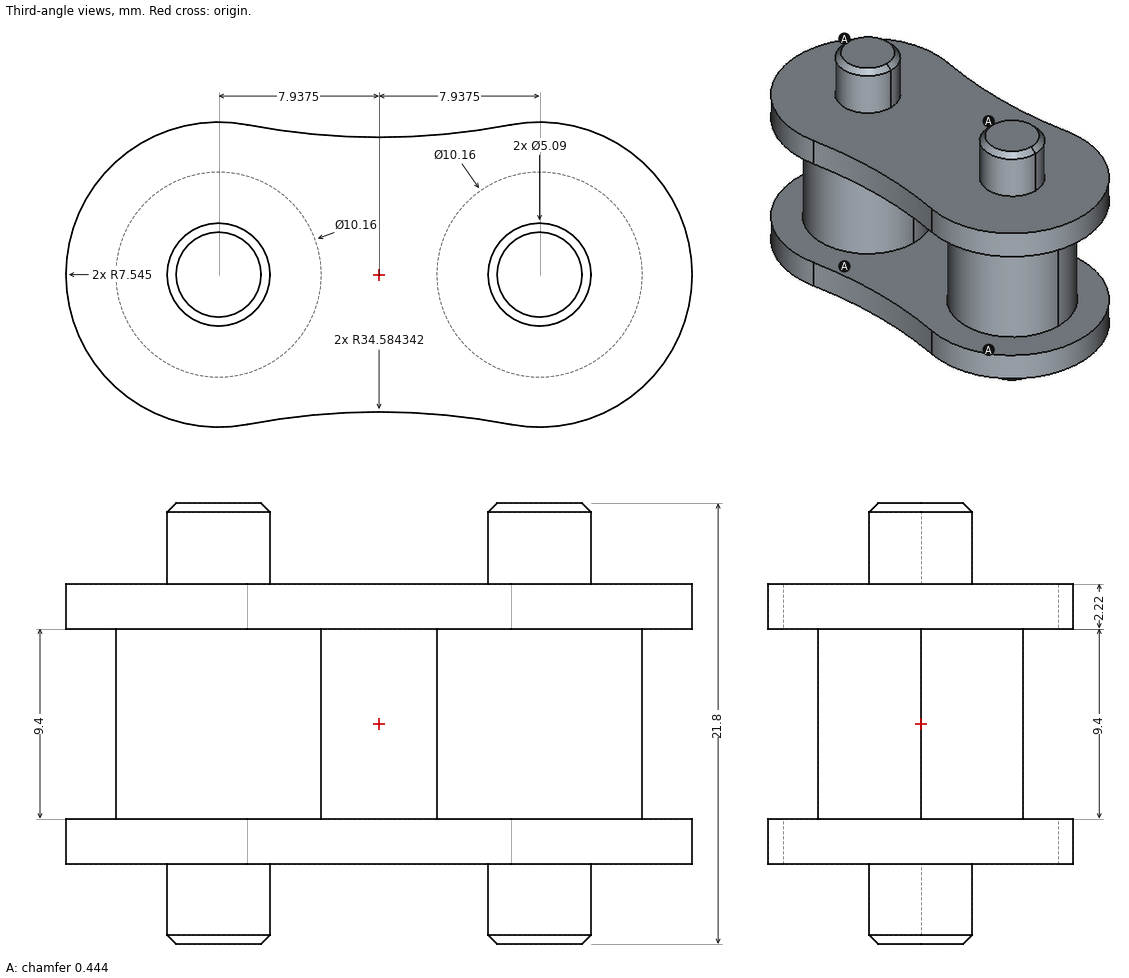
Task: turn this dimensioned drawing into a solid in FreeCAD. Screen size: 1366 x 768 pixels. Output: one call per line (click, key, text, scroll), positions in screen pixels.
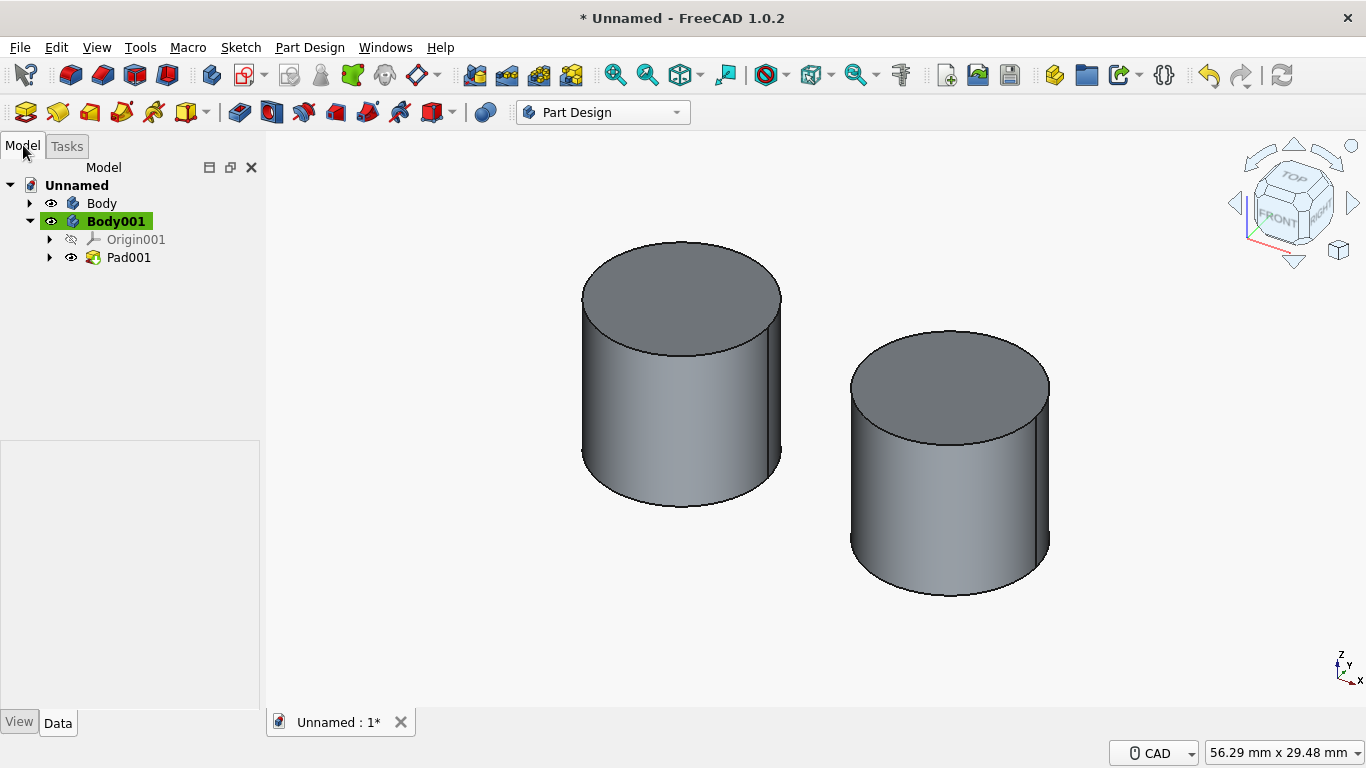
double_click(96, 203)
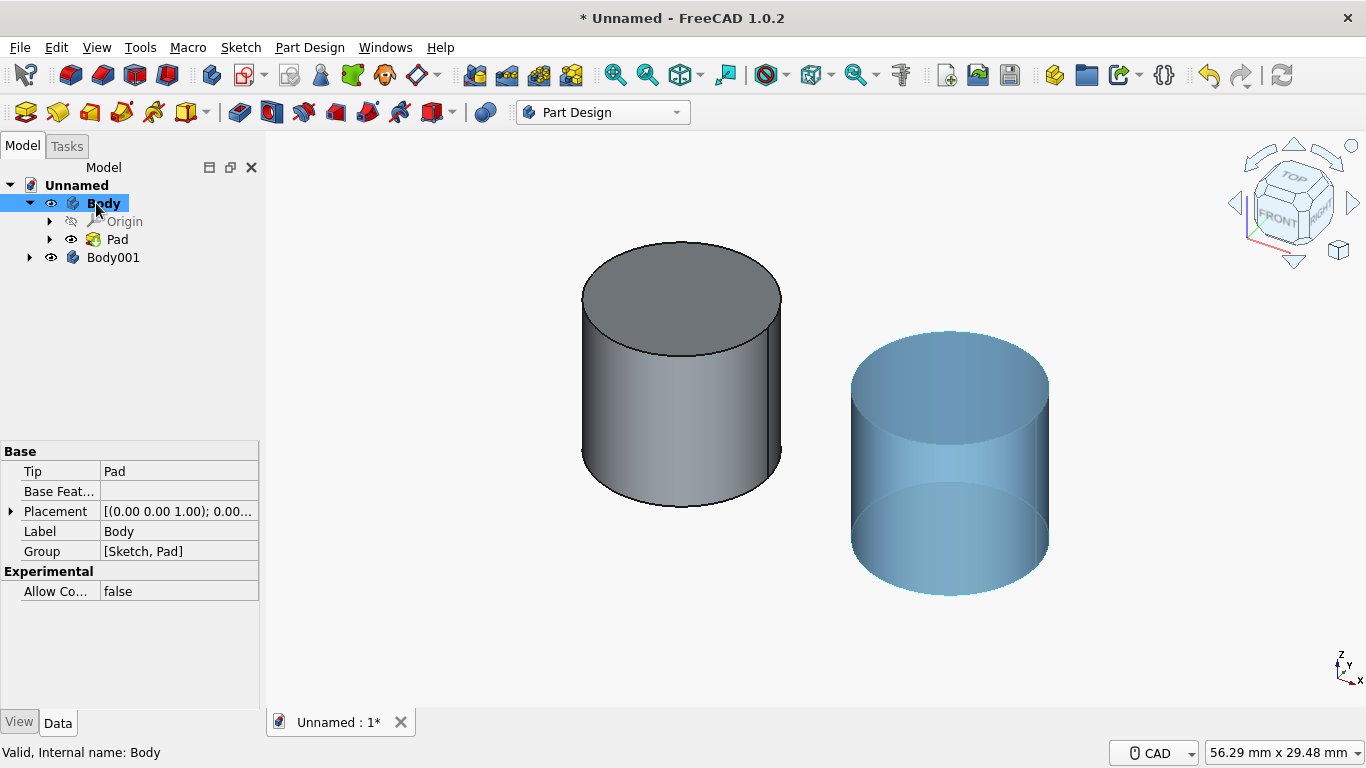
click(96, 203)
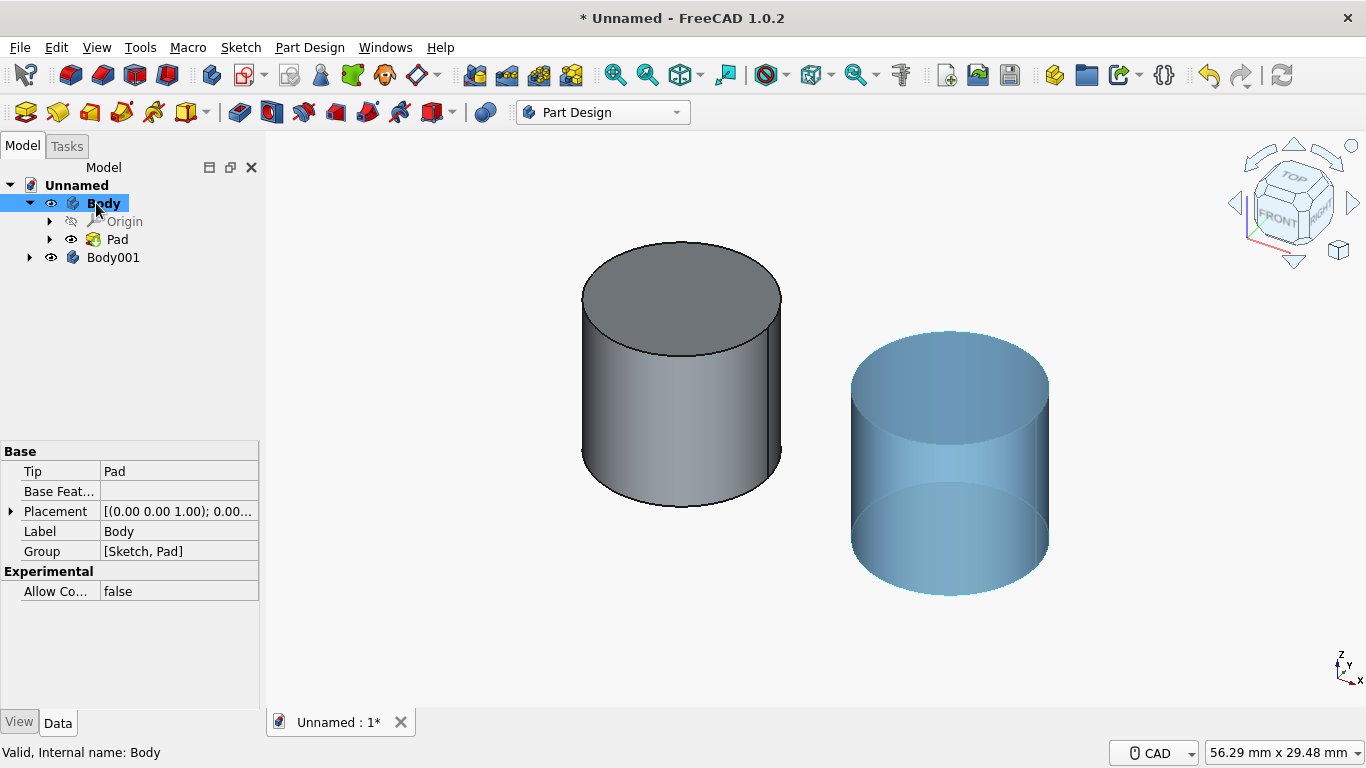
click(146, 591)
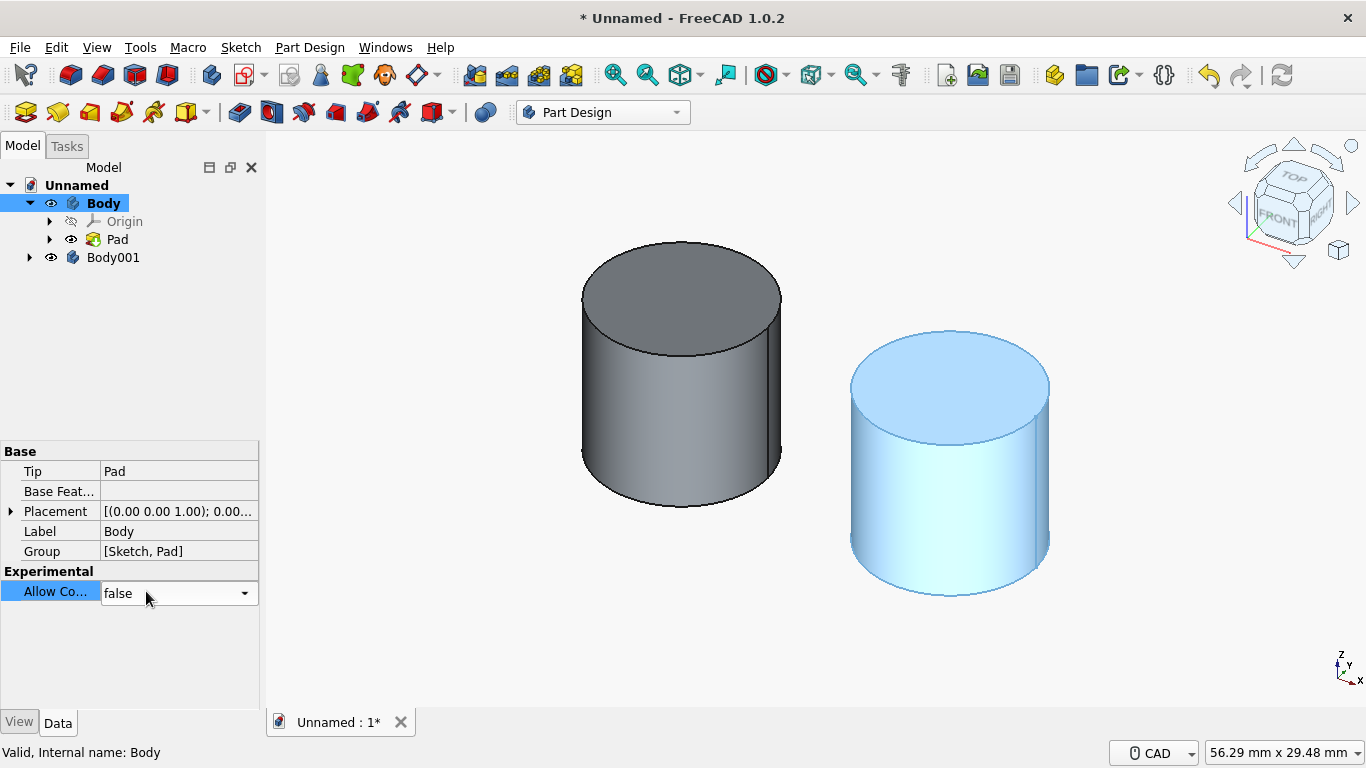
click(146, 591)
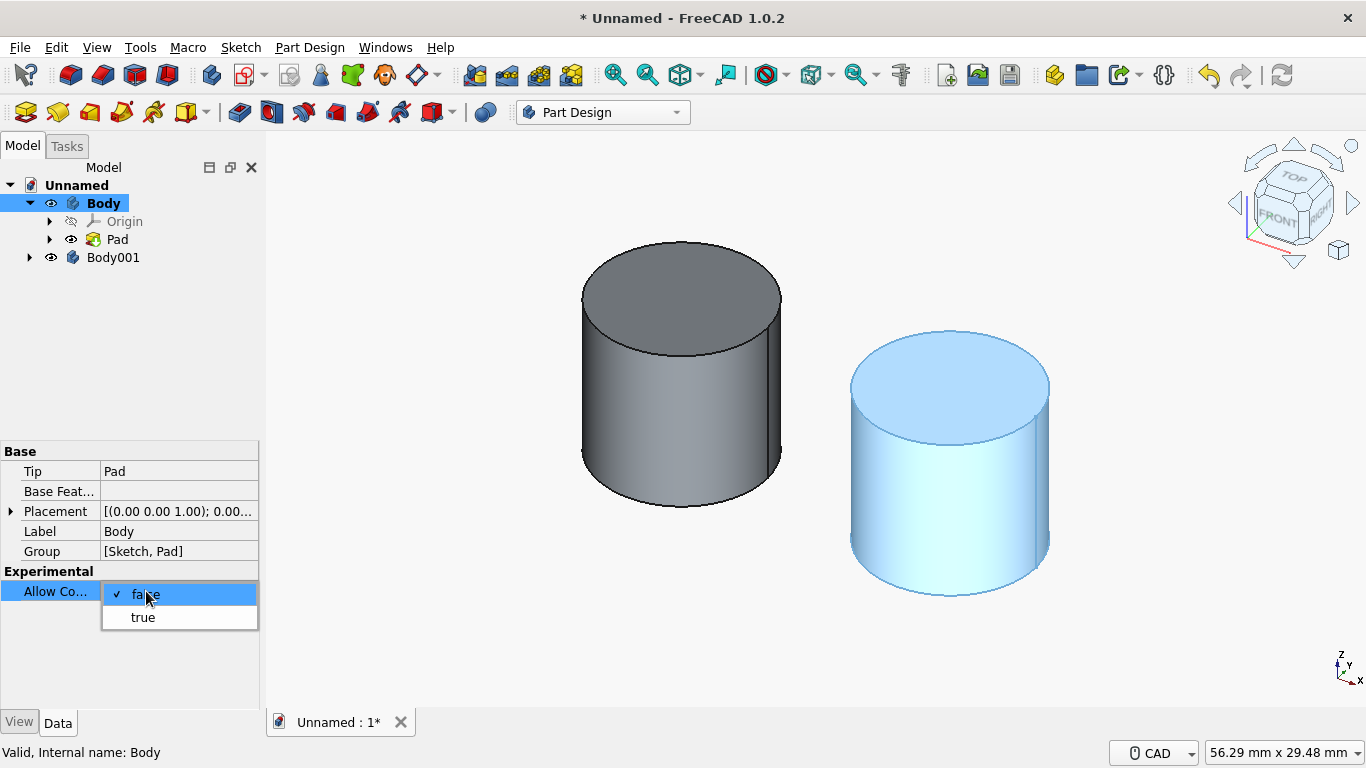
click(179, 618)
key(Return)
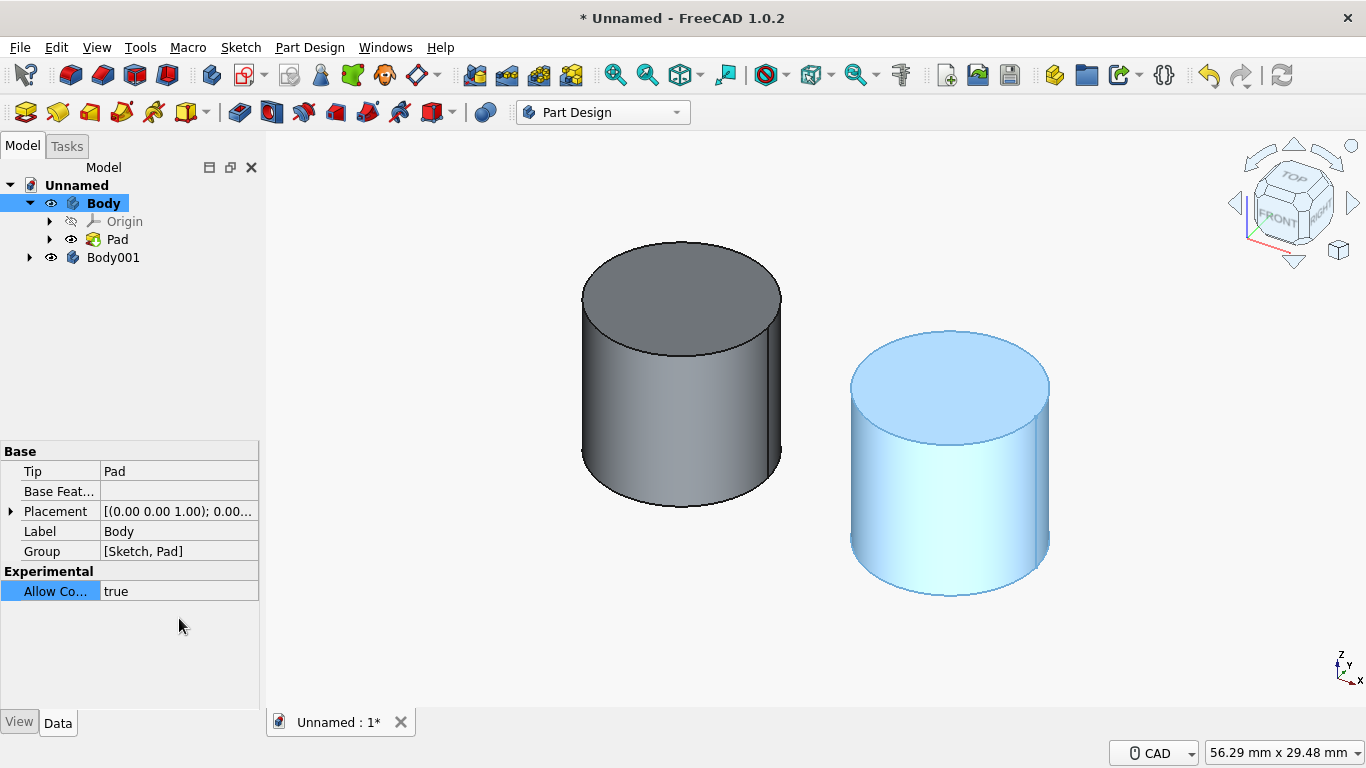
click(96, 257)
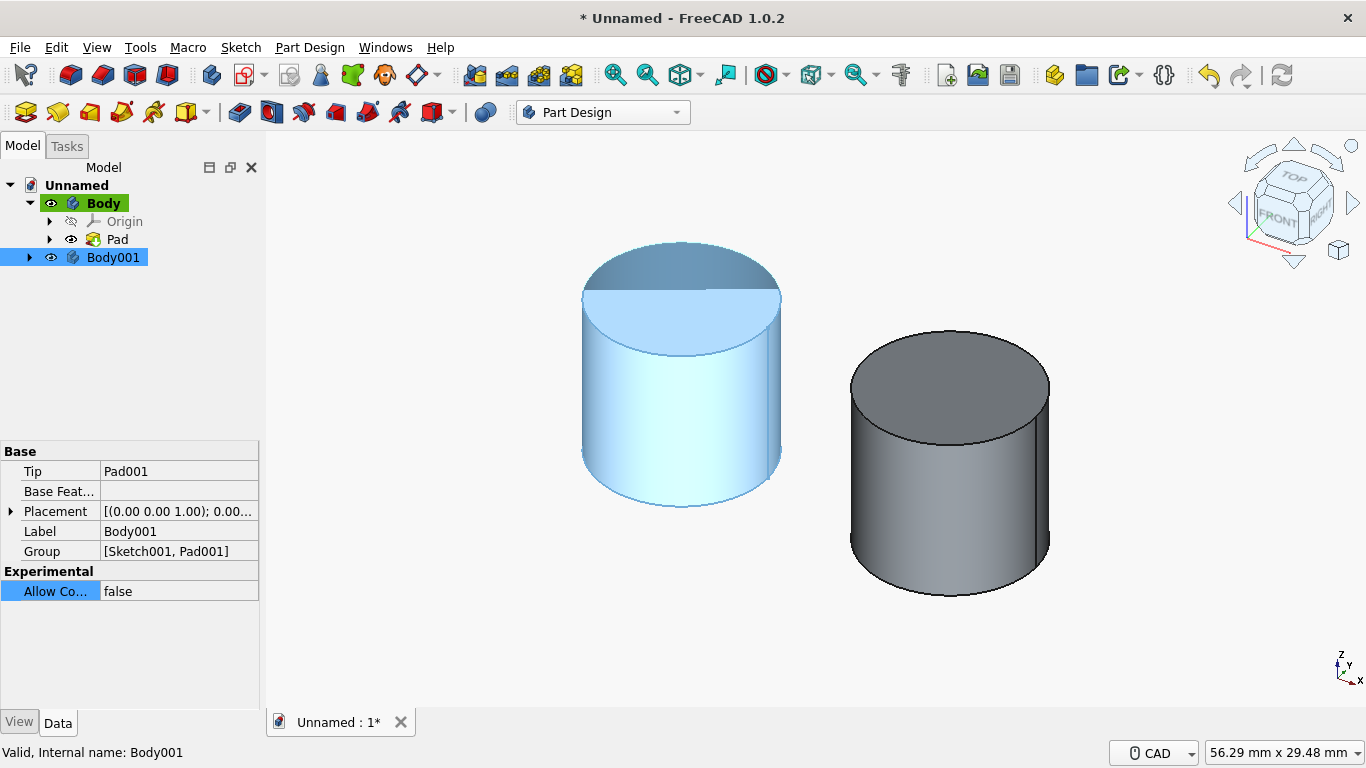
click(486, 112)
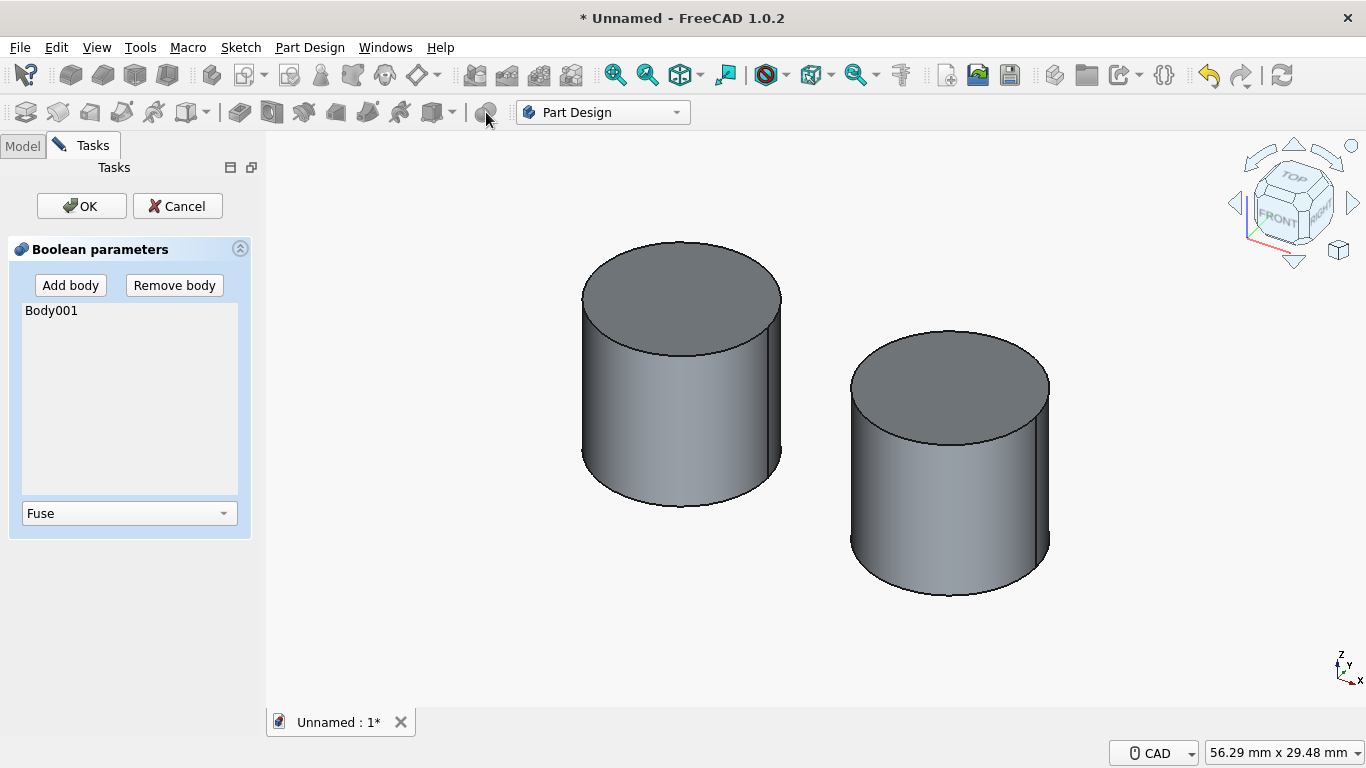
click(82, 206)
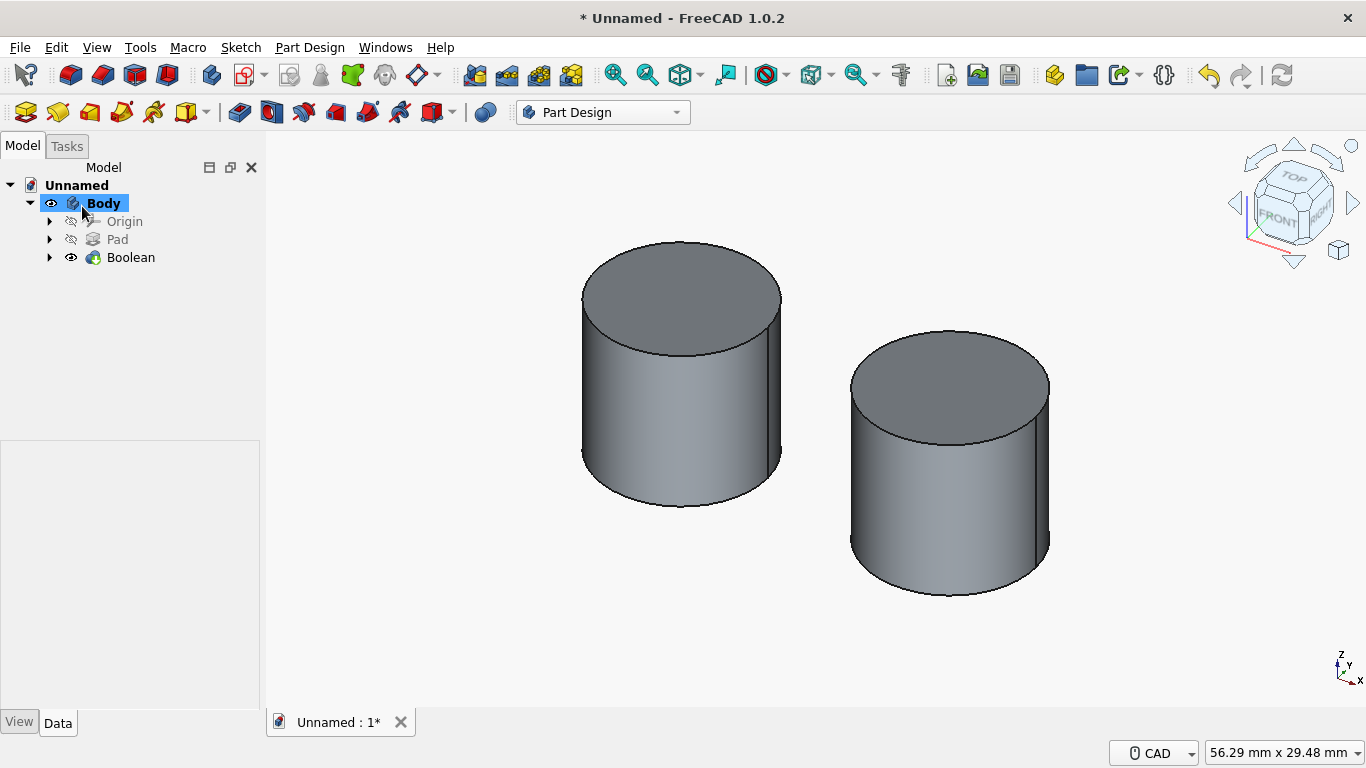
click(682, 298)